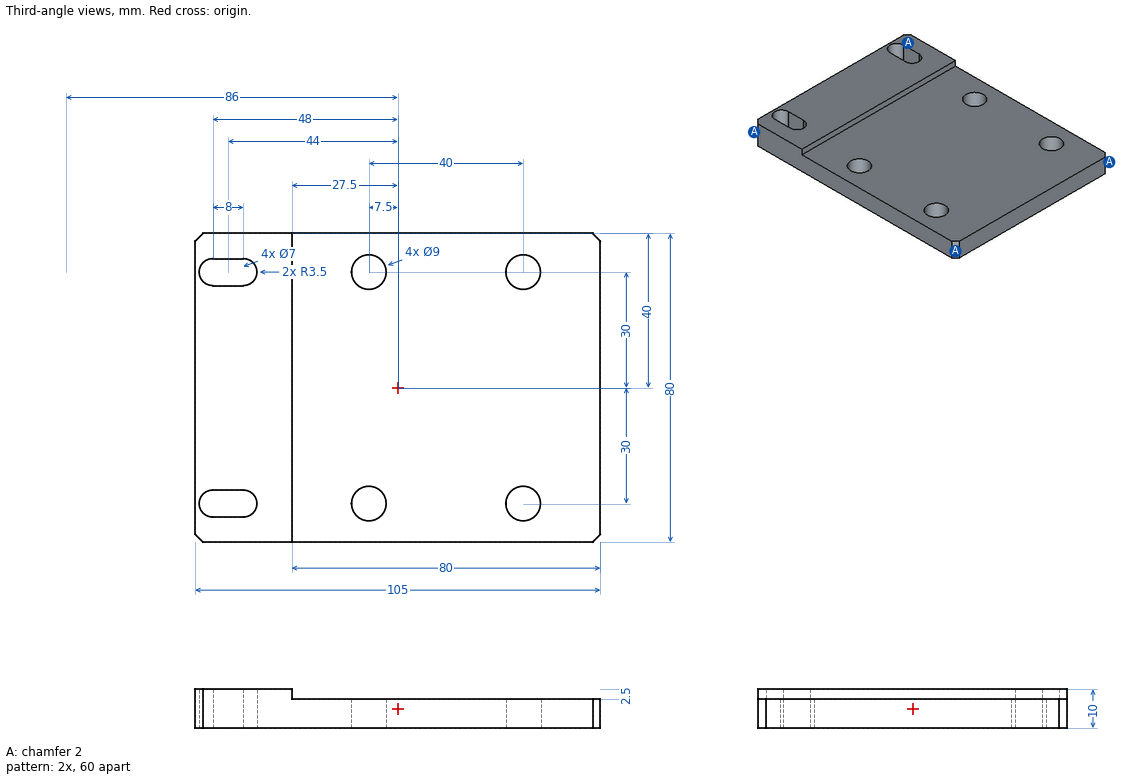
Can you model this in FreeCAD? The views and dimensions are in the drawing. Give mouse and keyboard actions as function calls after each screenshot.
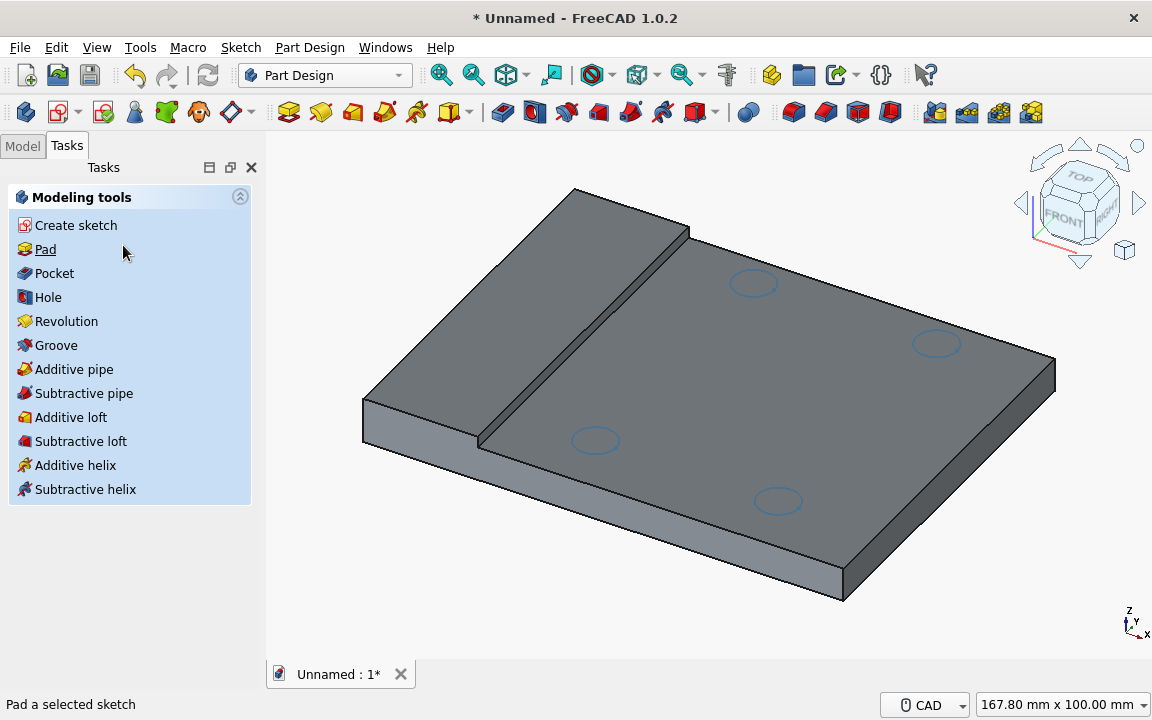
click(504, 112)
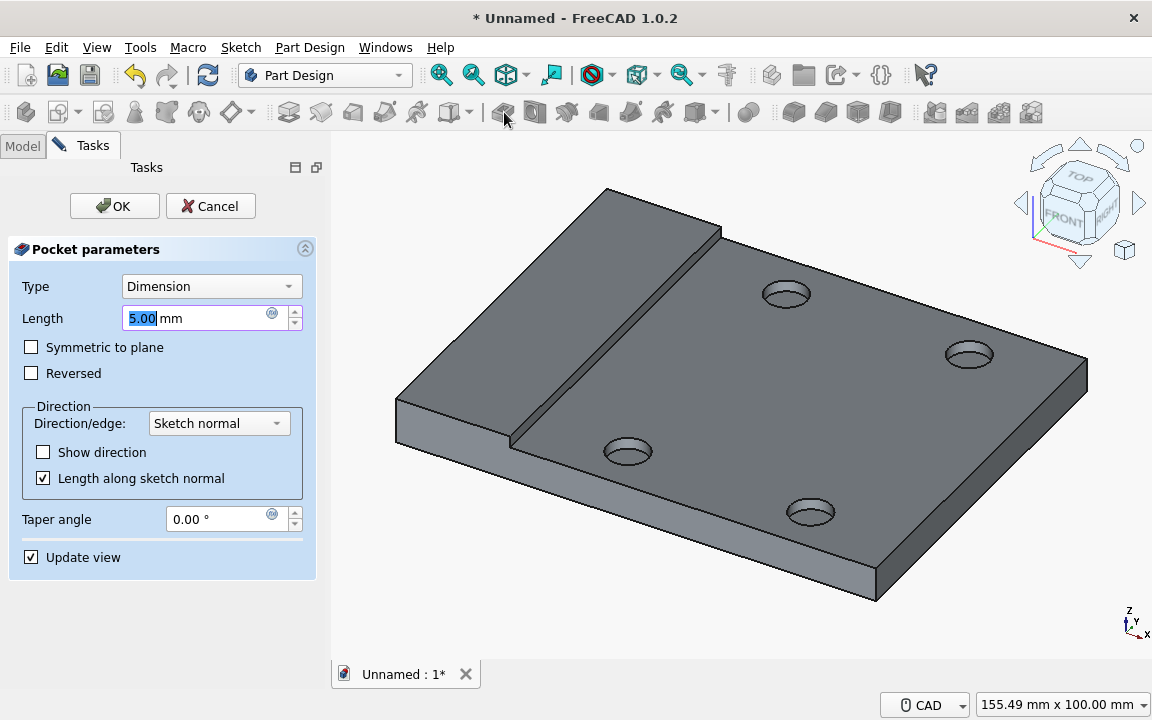
click(212, 286)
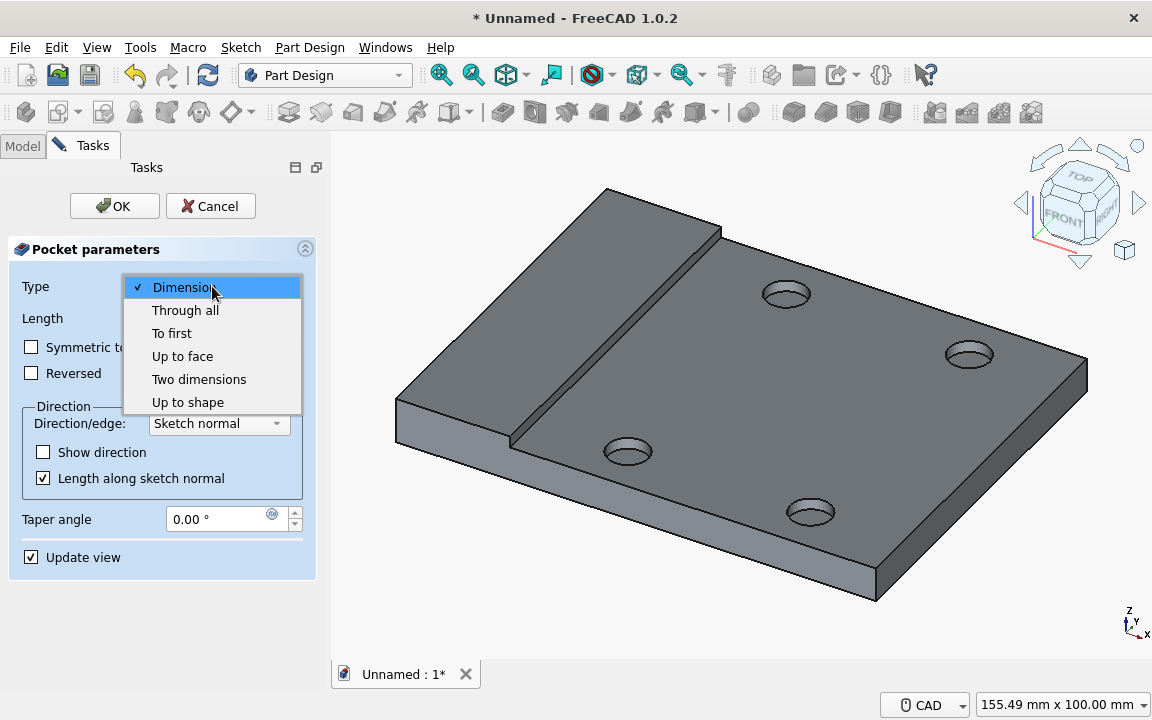
click(212, 310)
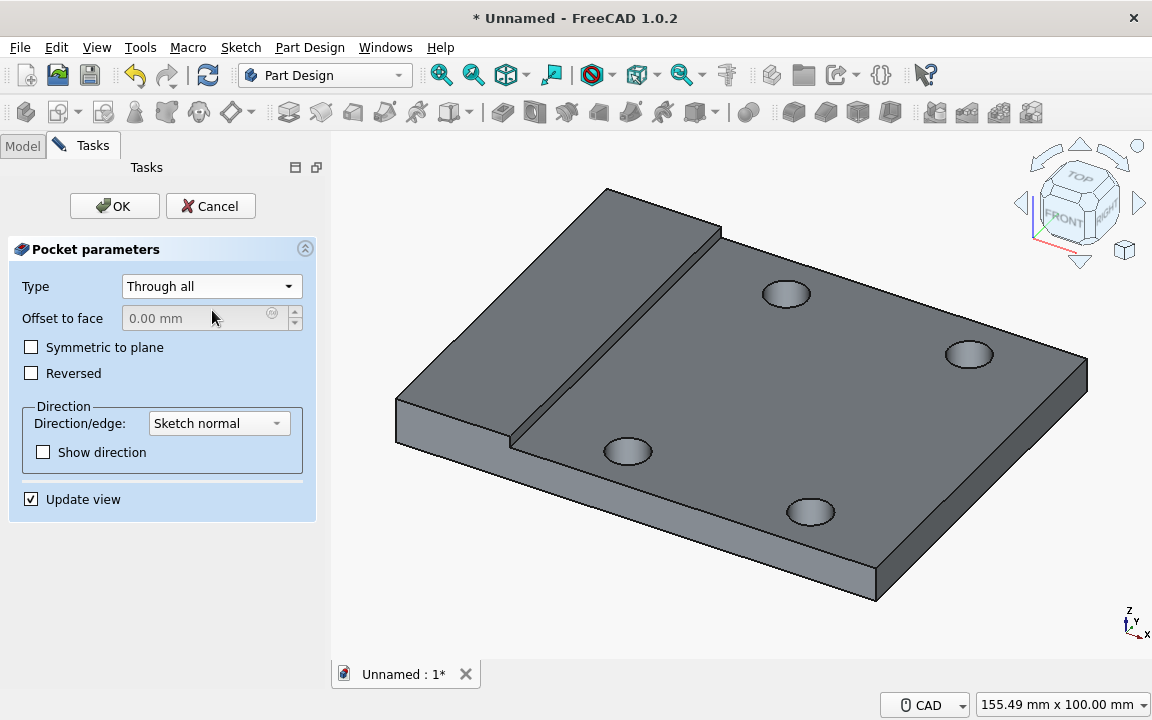
click(115, 206)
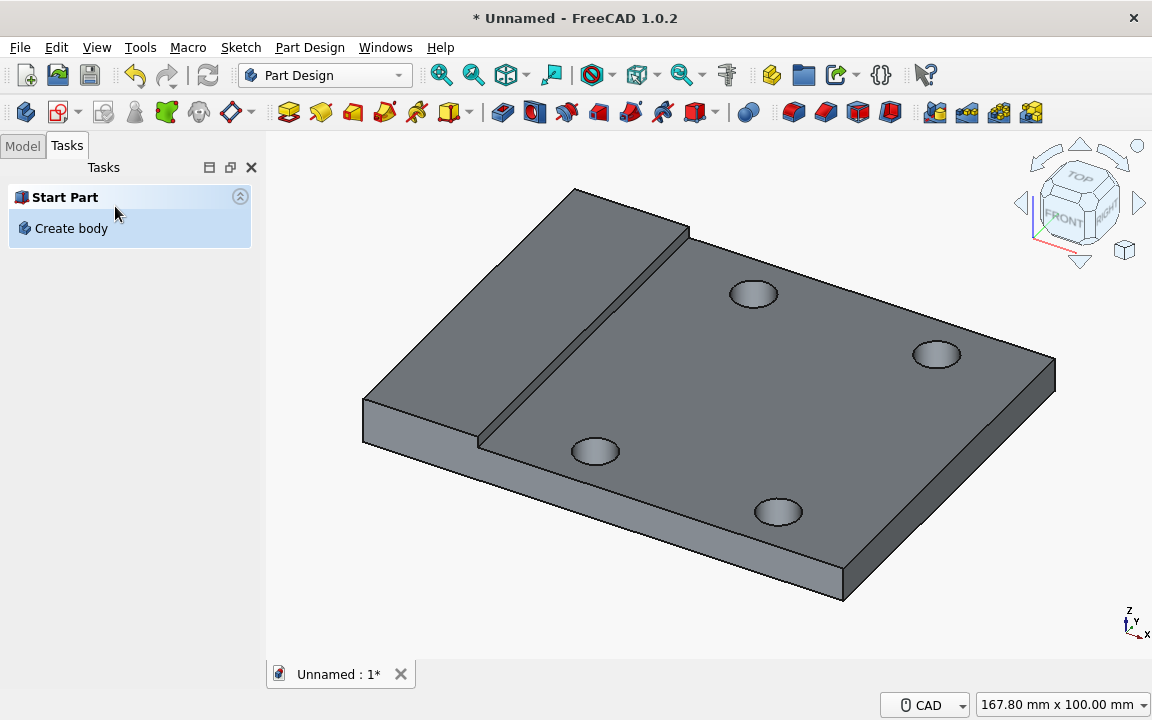
click(586, 252)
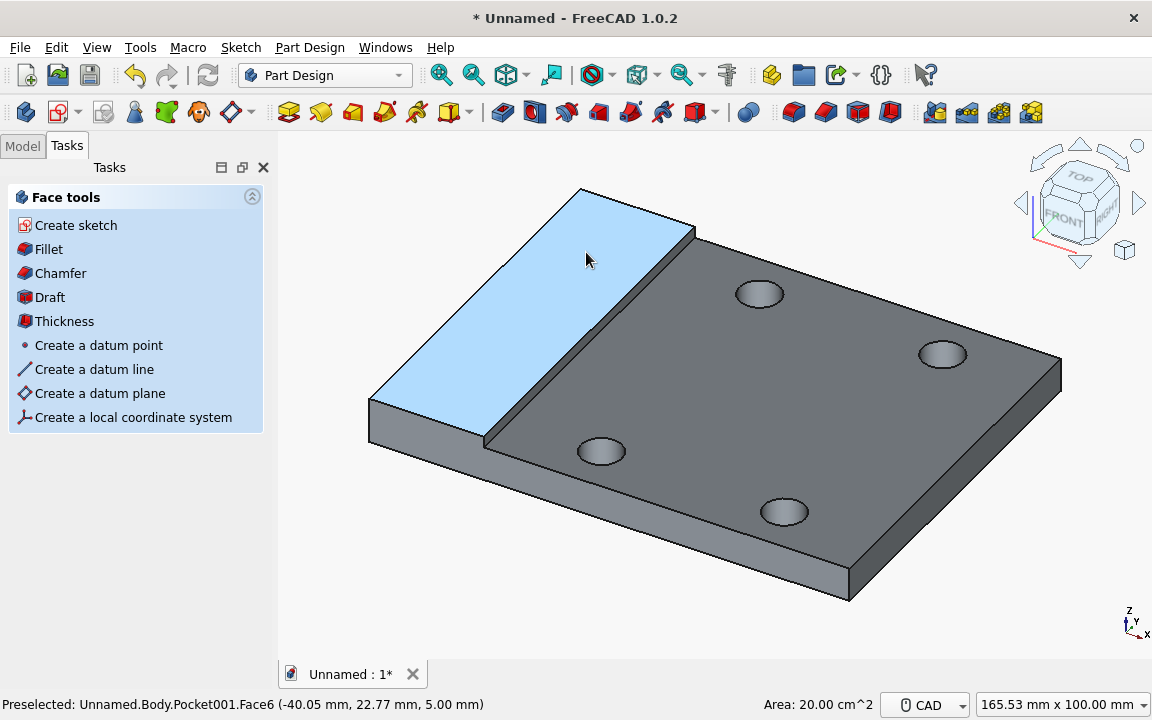
click(58, 112)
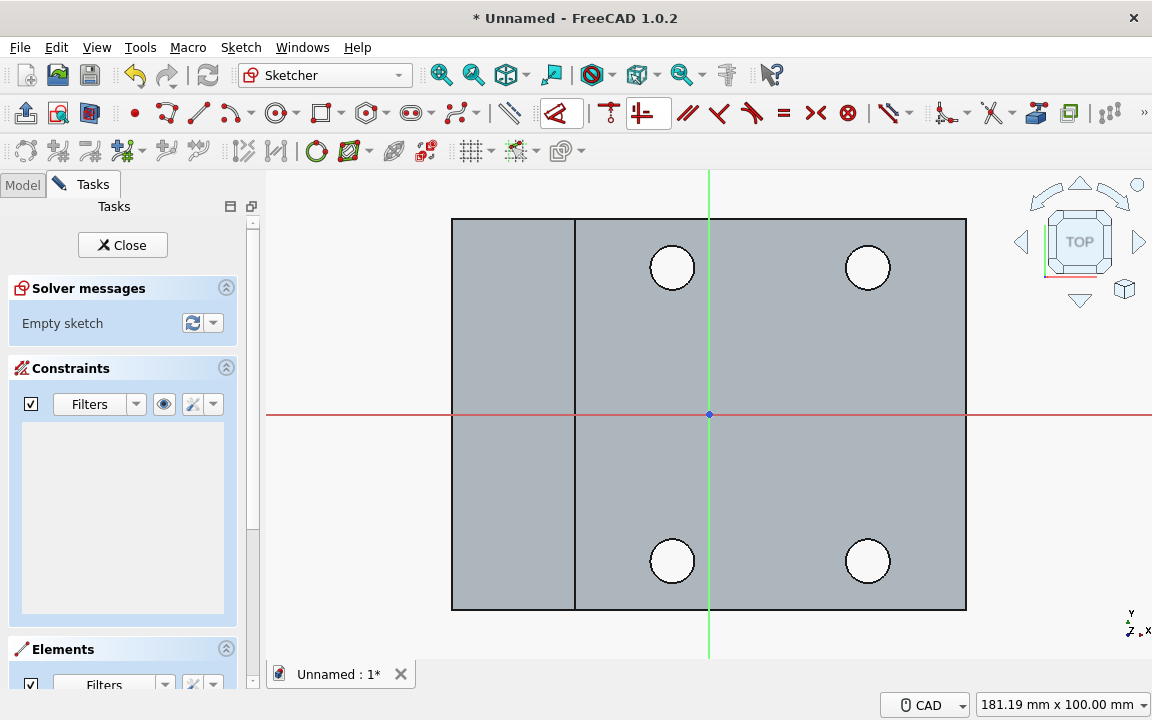
scroll(987, 415, down, 1)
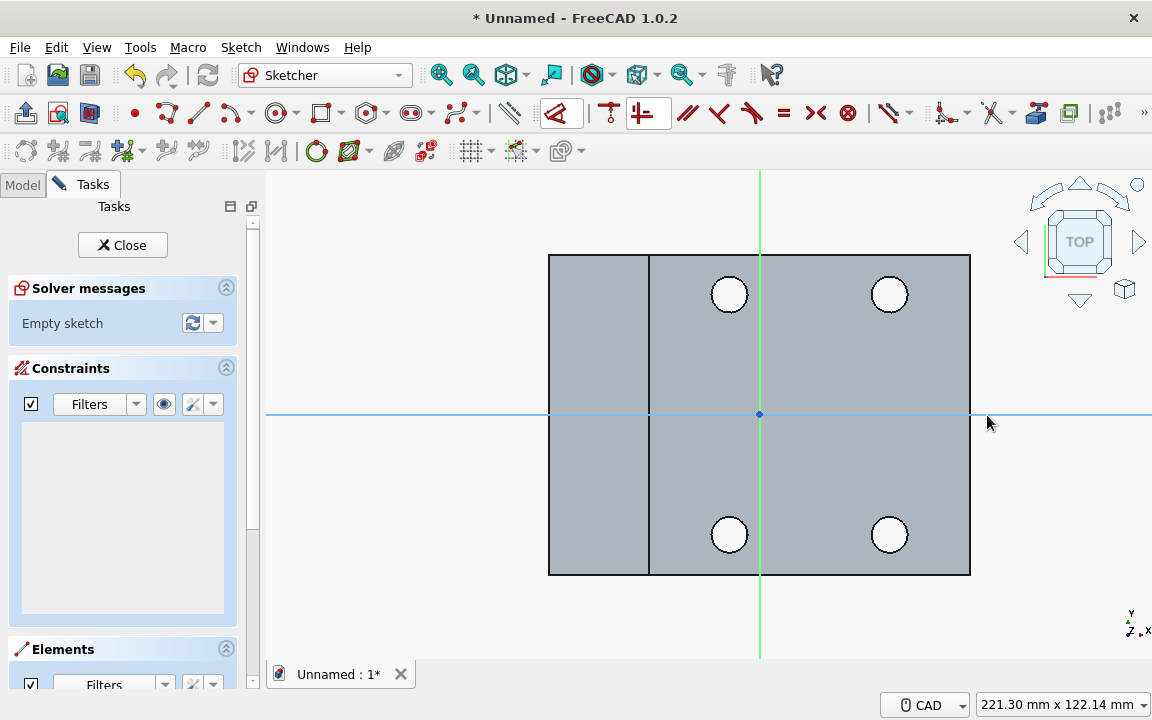
click(276, 114)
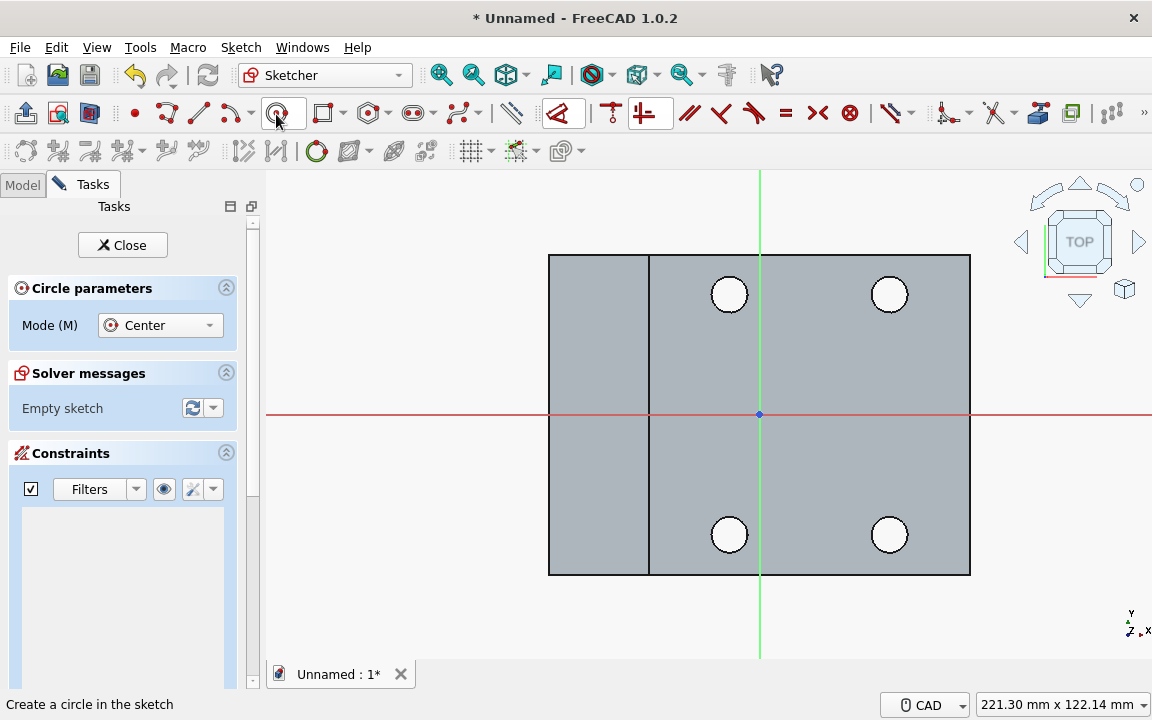
scroll(583, 295, up, 3)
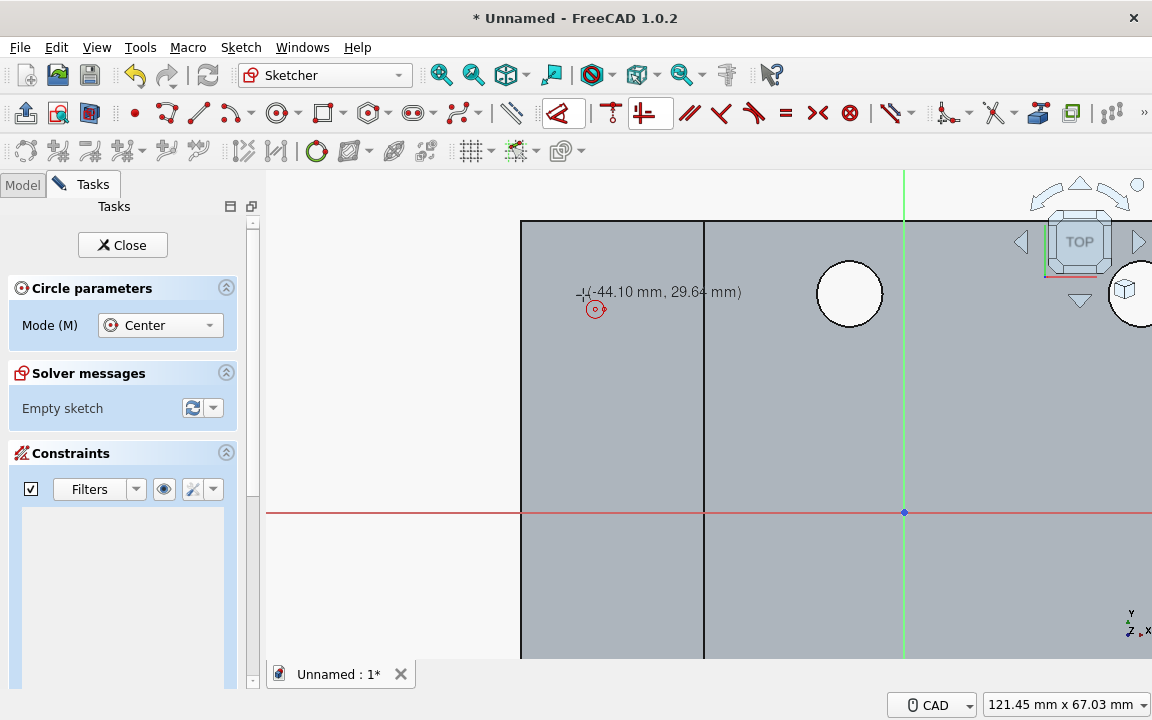
click(583, 294)
click(601, 276)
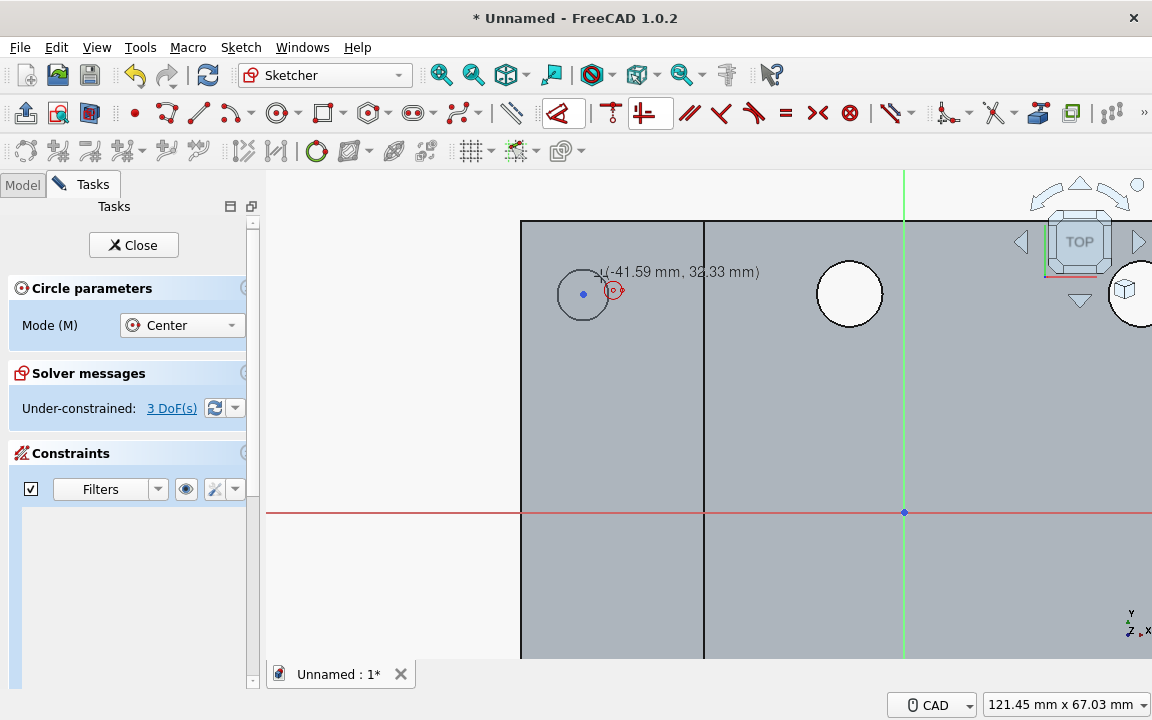
scroll(768, 215, down, 2)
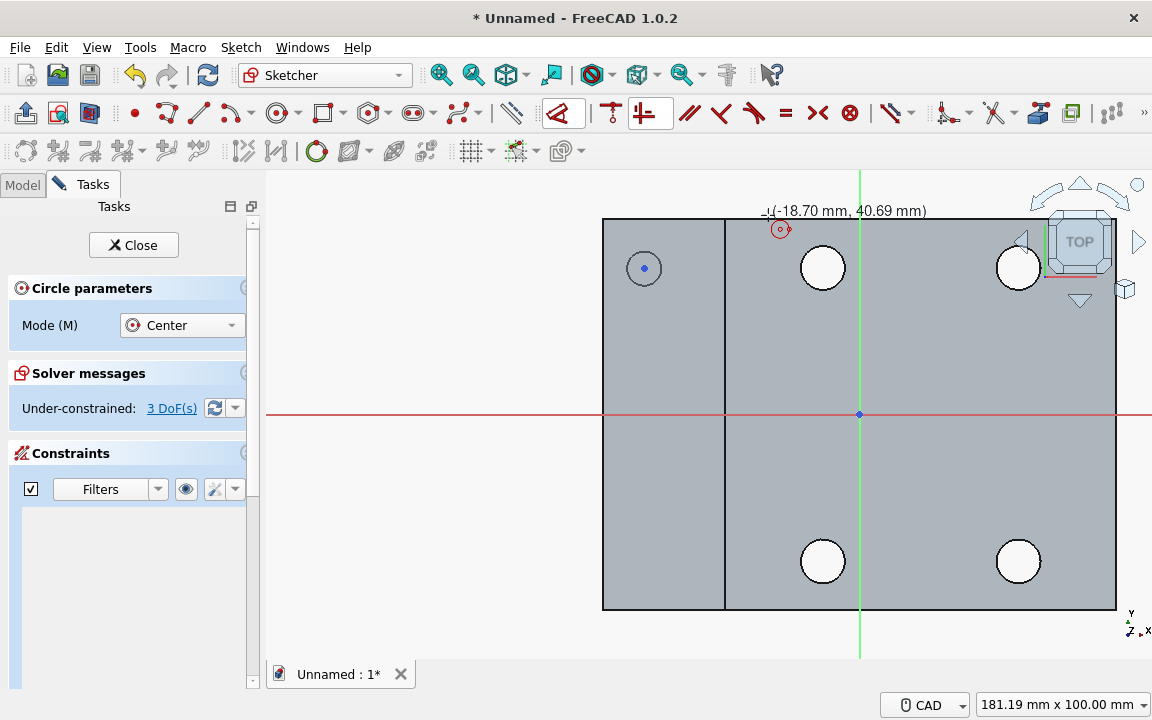
scroll(439, 268, up, 2)